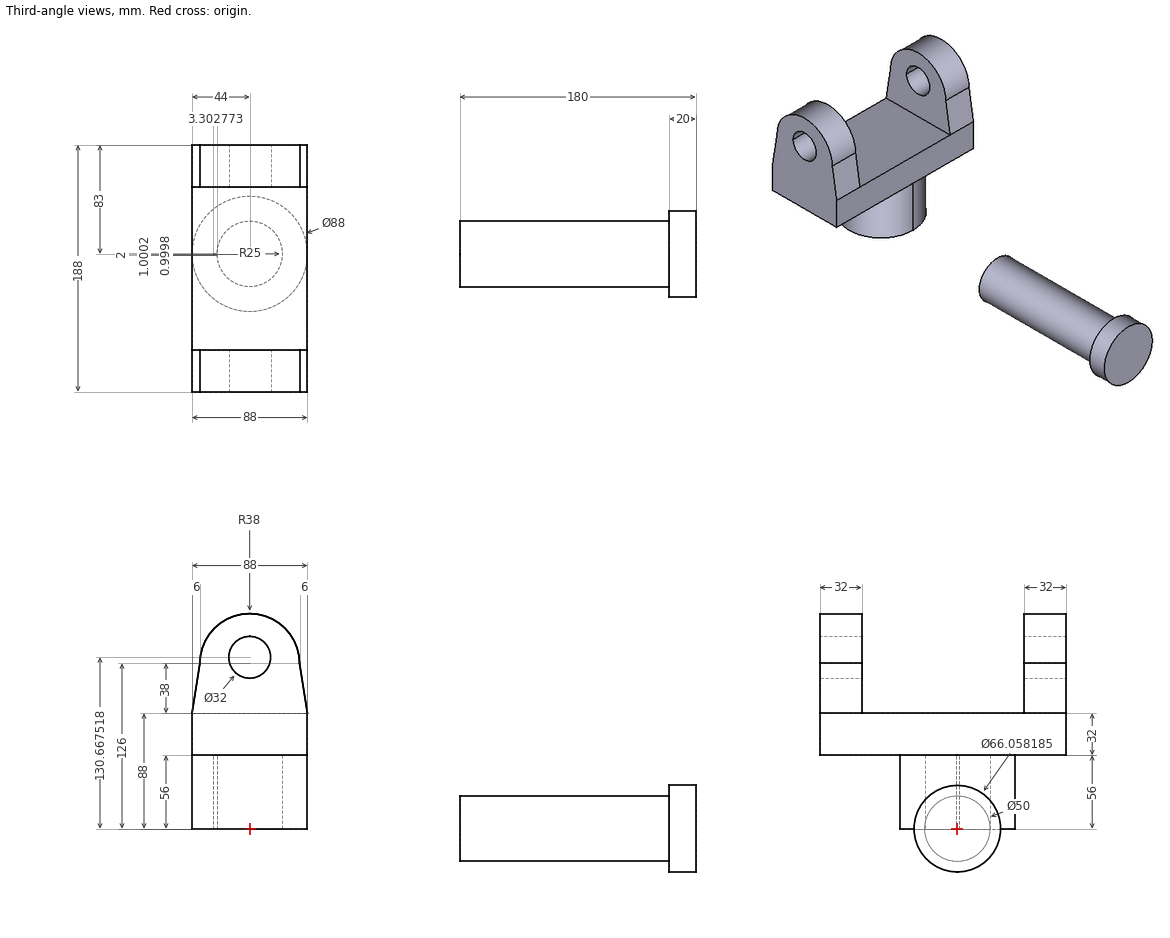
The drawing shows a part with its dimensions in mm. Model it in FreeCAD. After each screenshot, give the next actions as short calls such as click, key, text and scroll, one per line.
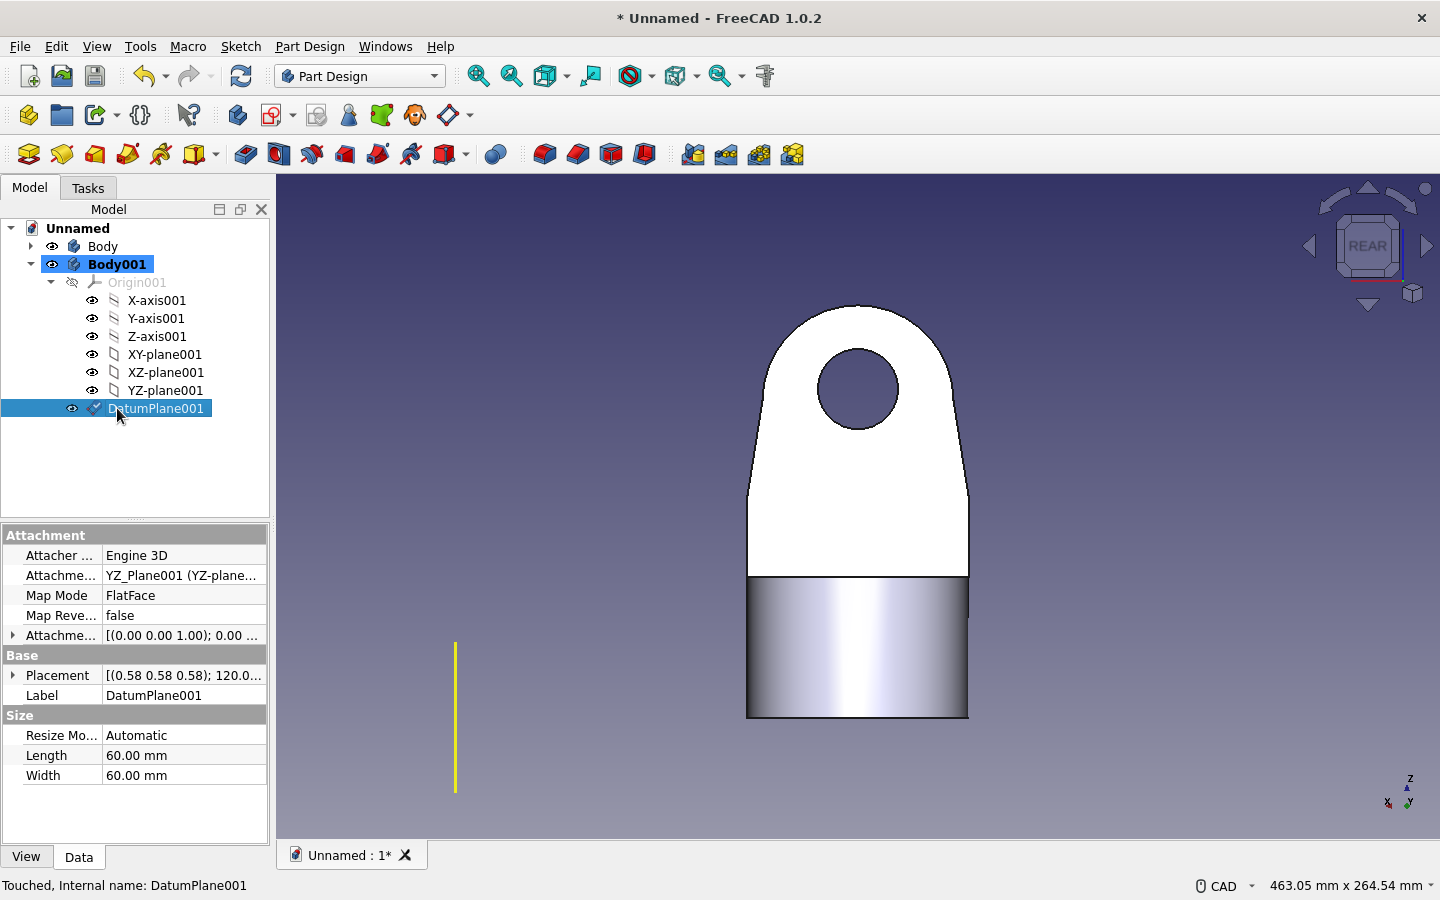
click(270, 116)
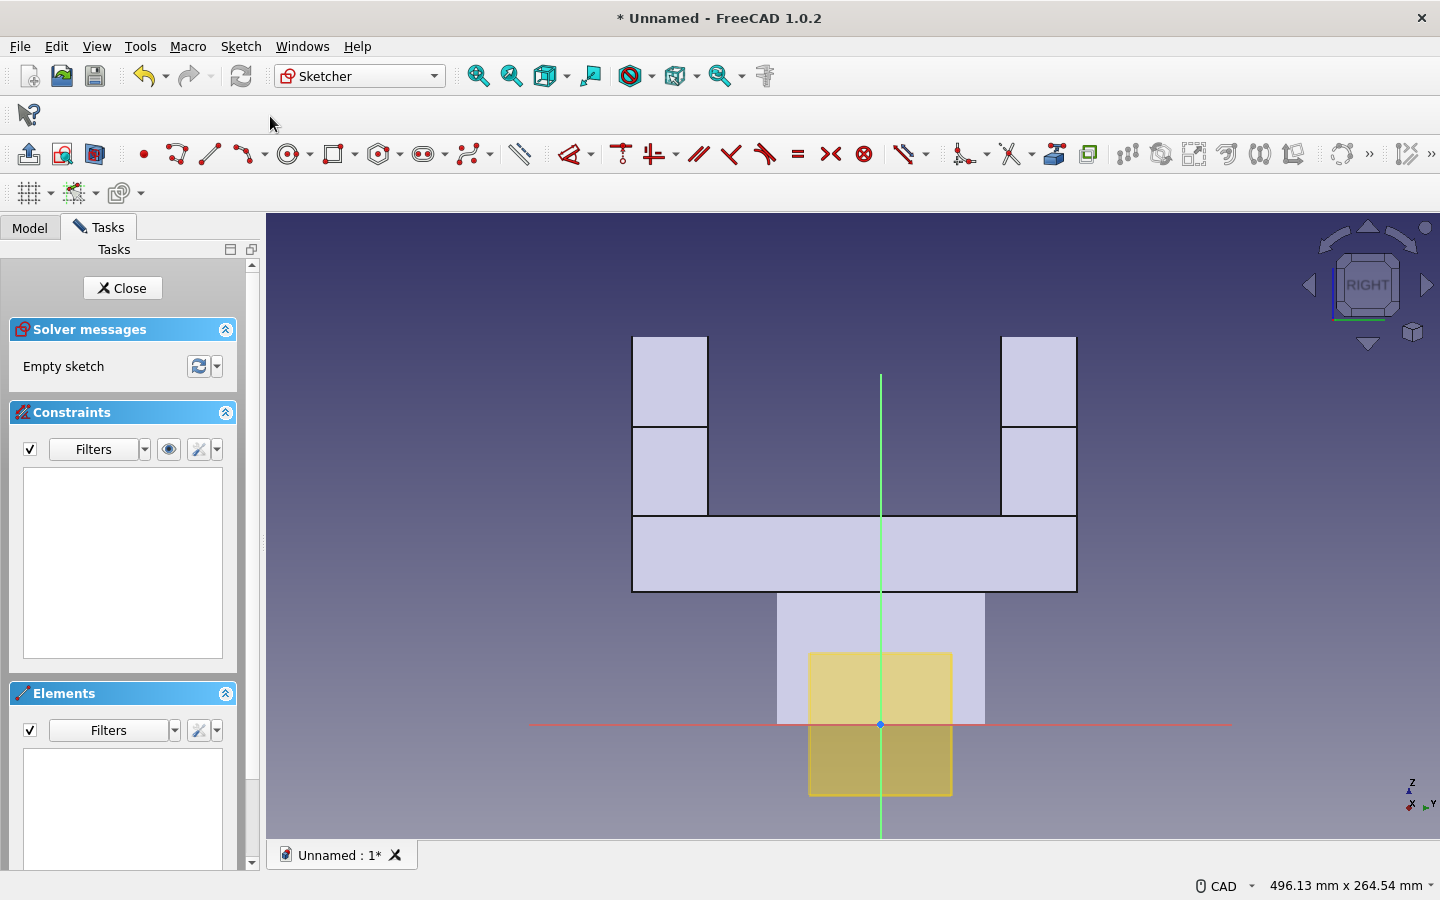
scroll(922, 810, up, 6)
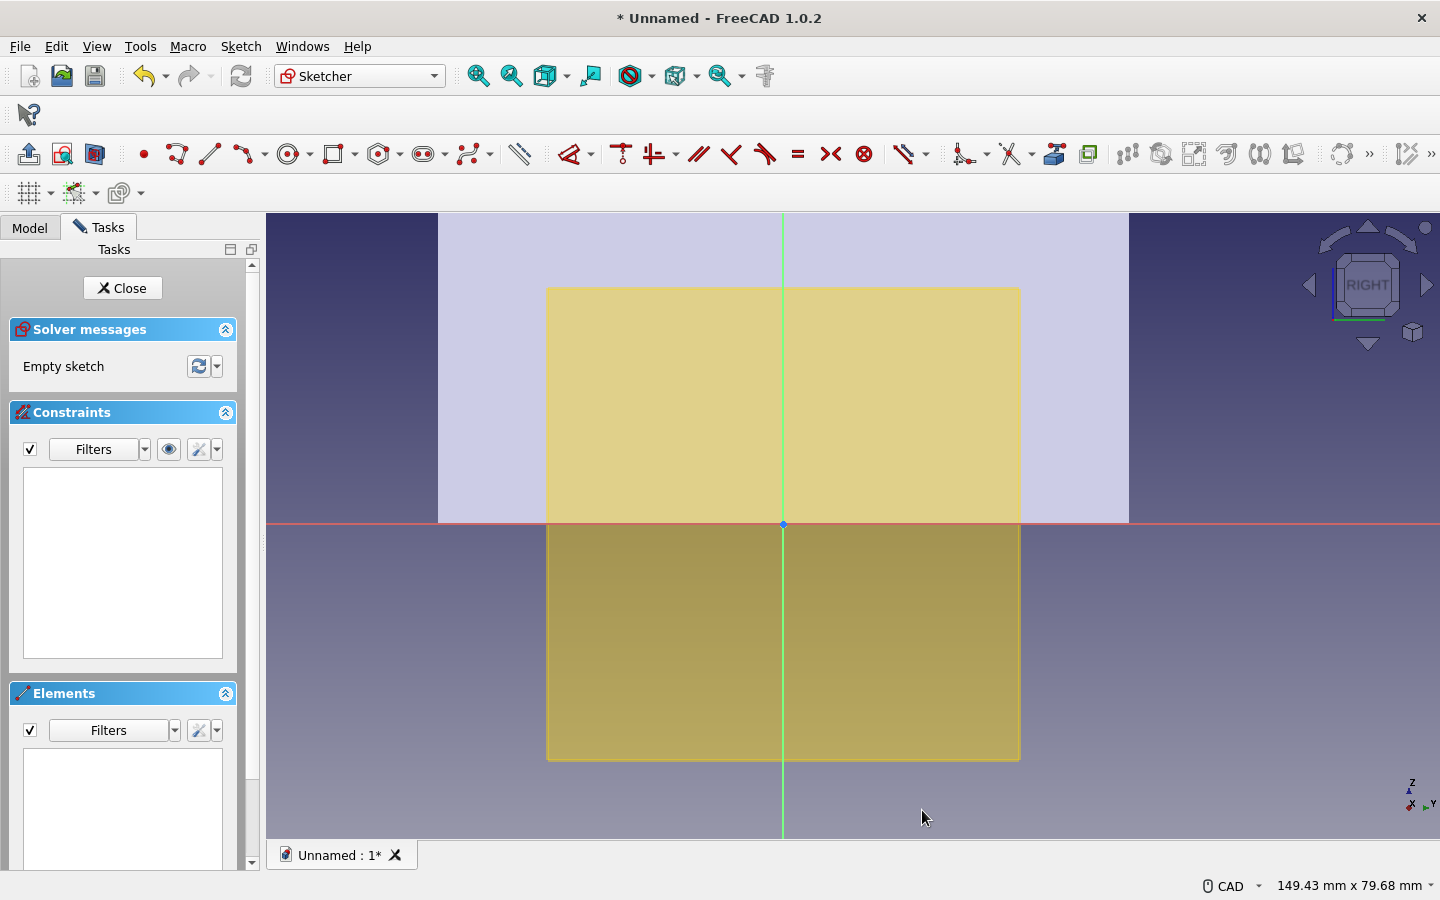
key(g)
key(c)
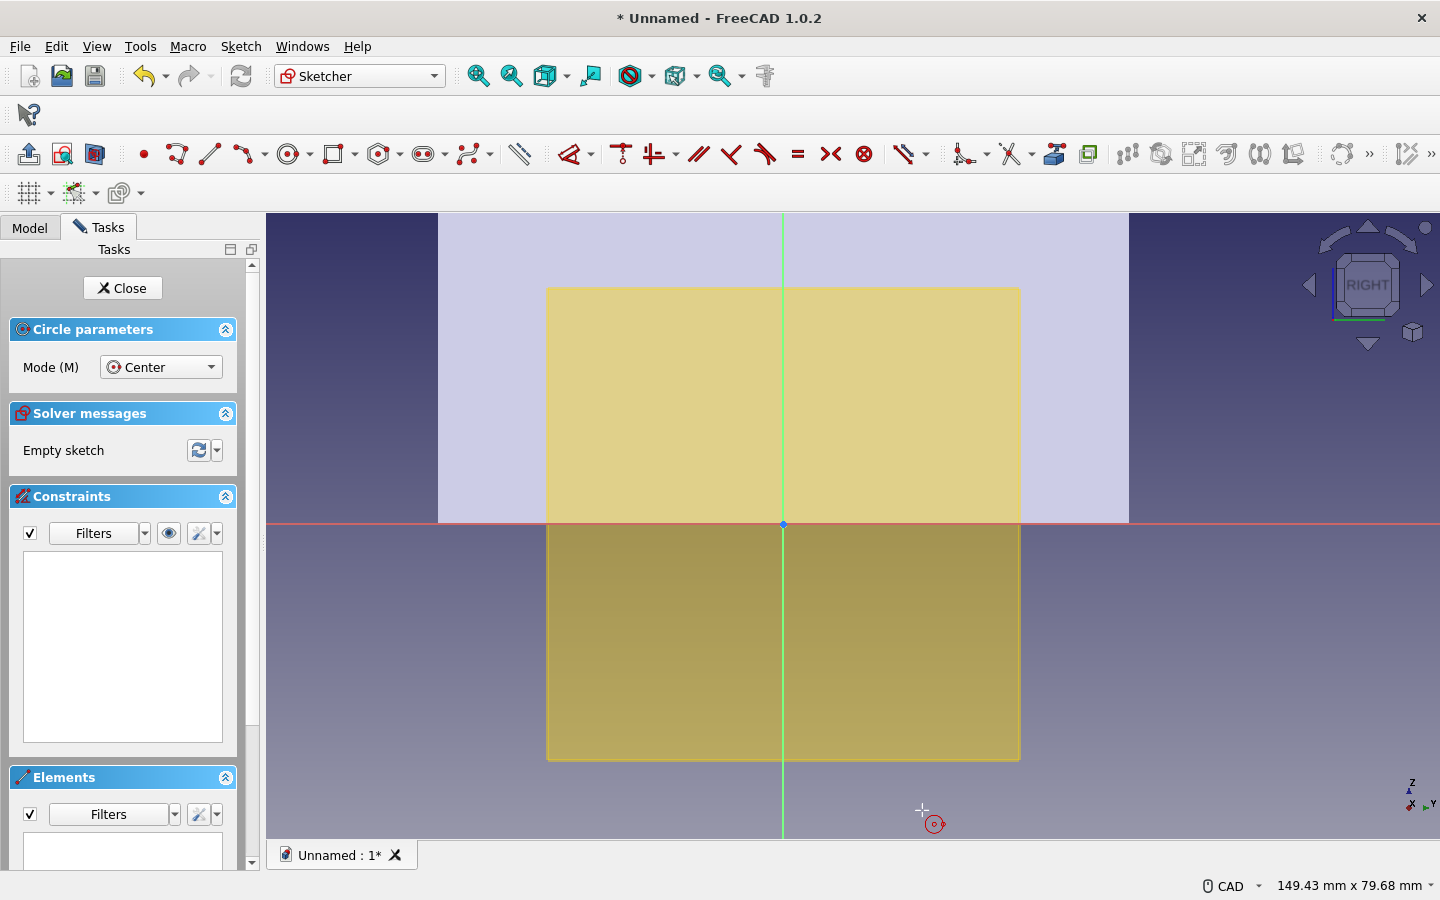
click(783, 524)
click(922, 386)
key(Escape)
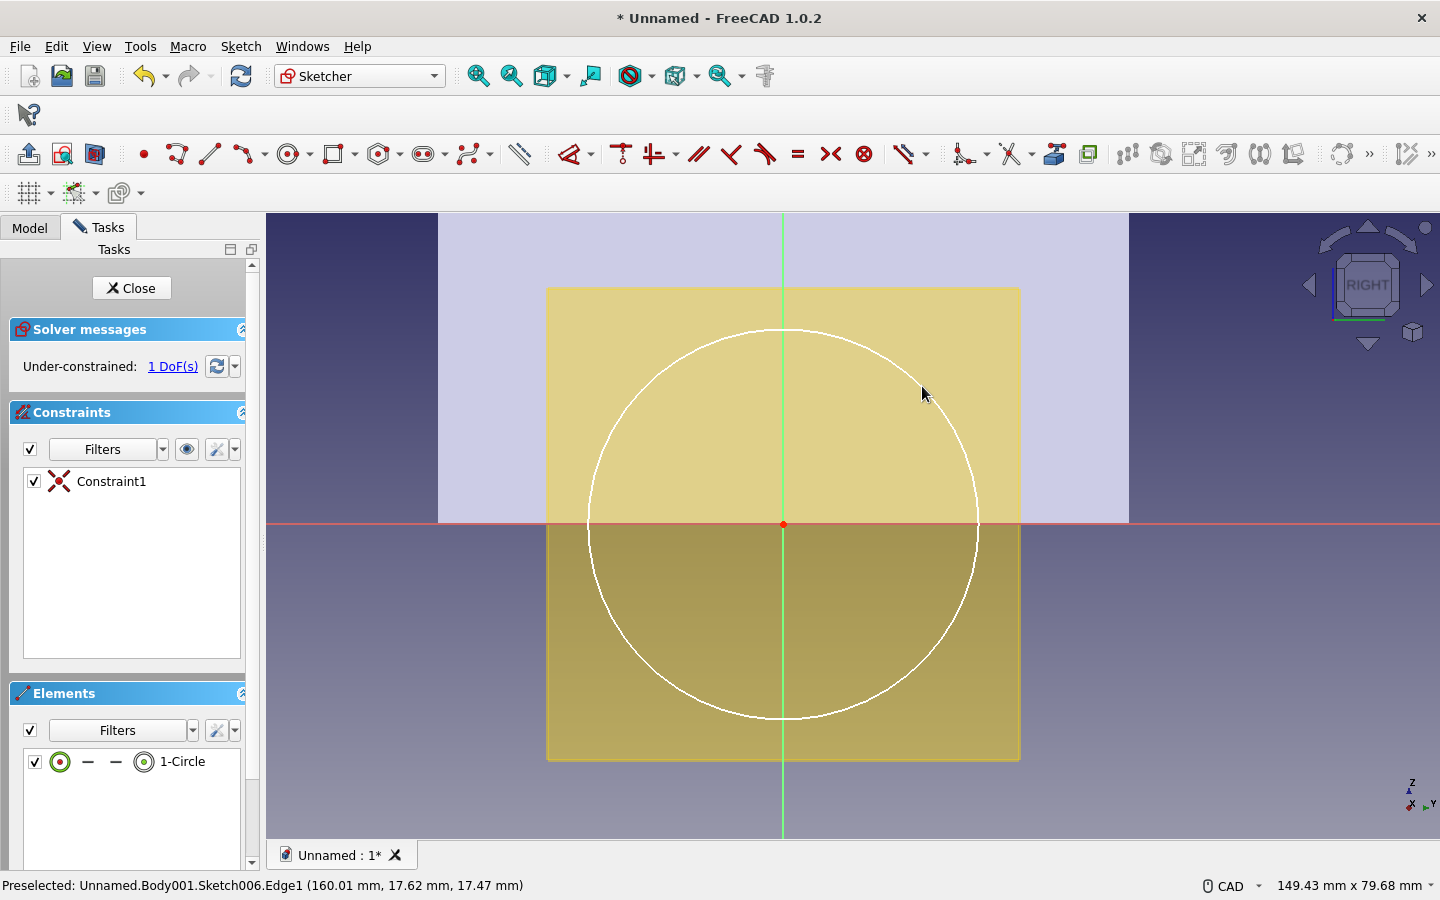
key(d)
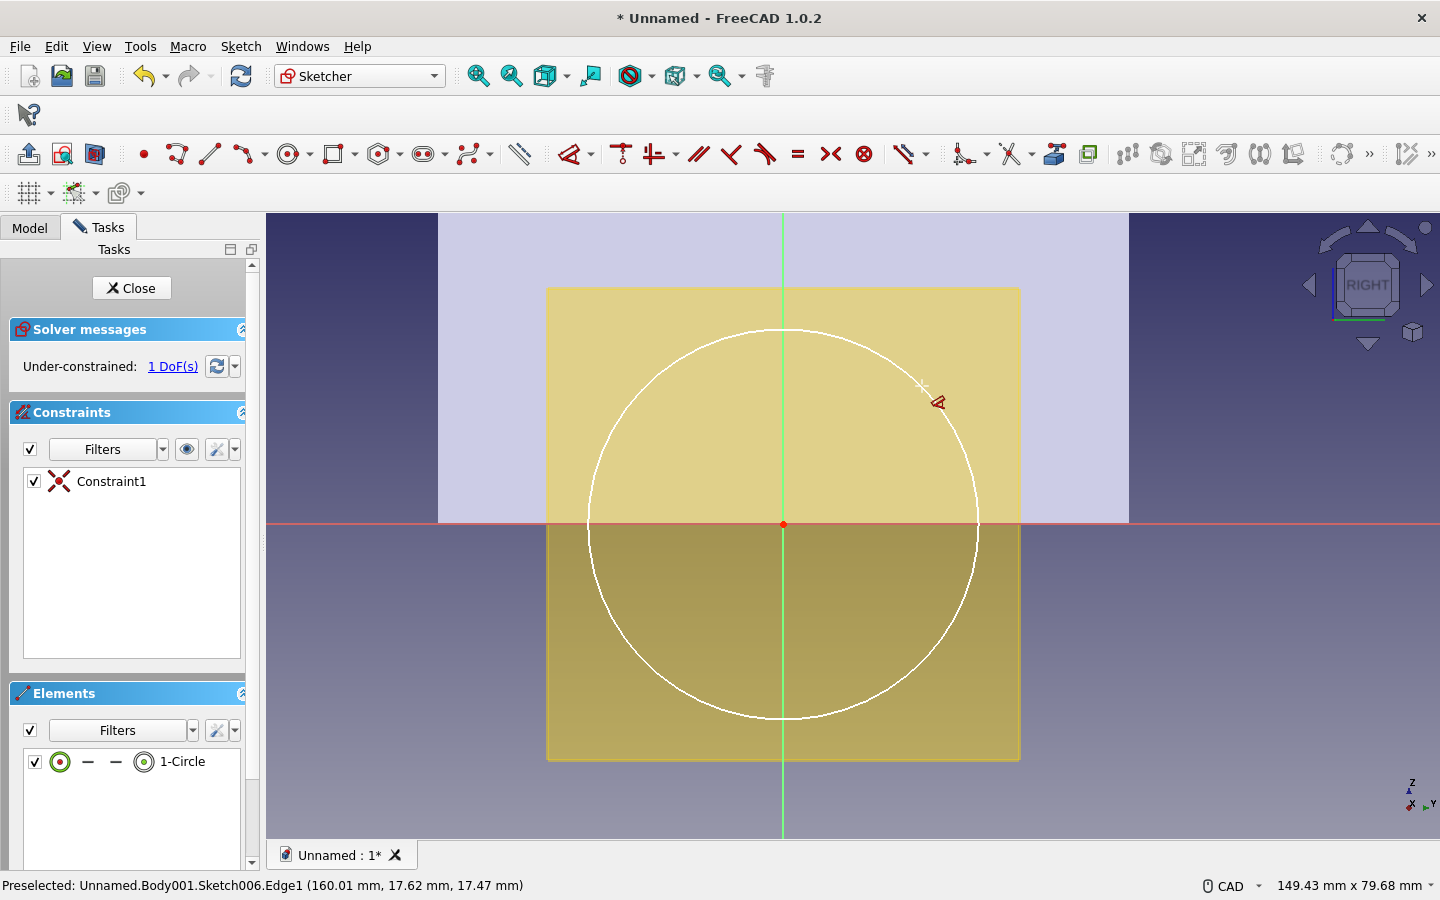
click(921, 386)
click(944, 363)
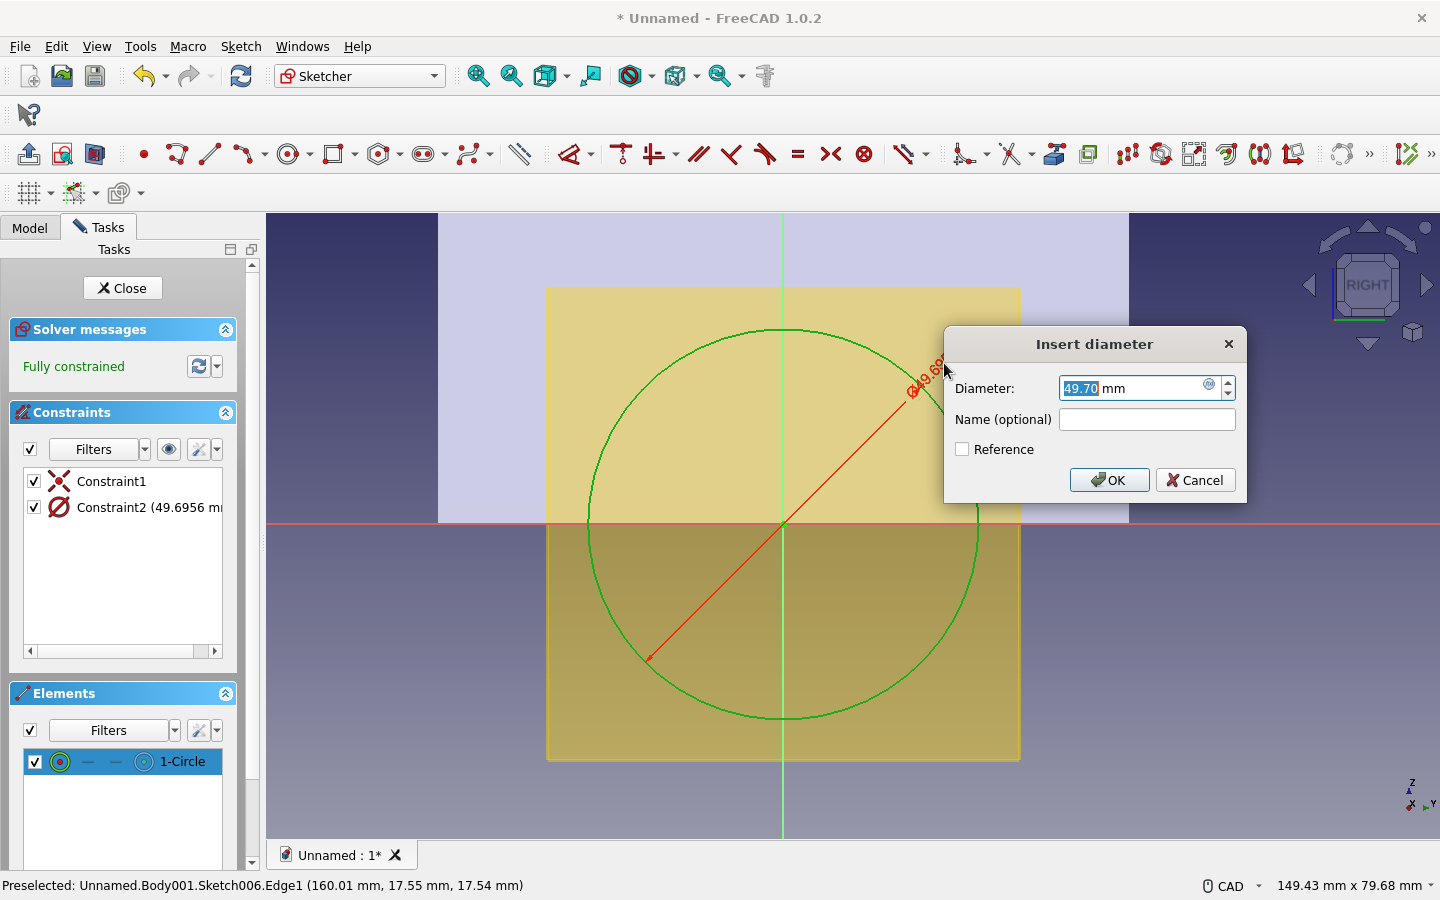
text(50)
key(Return)
key(Escape)